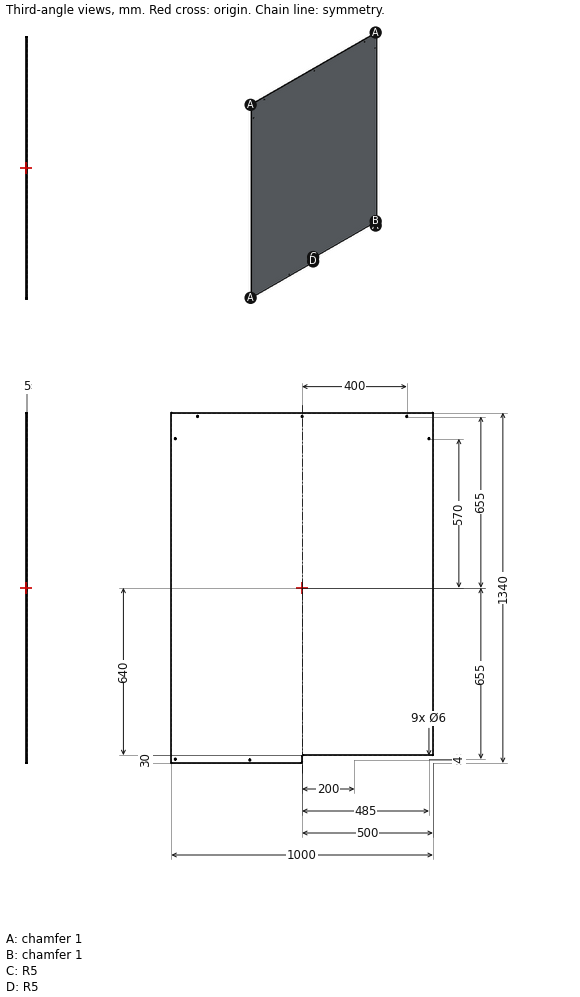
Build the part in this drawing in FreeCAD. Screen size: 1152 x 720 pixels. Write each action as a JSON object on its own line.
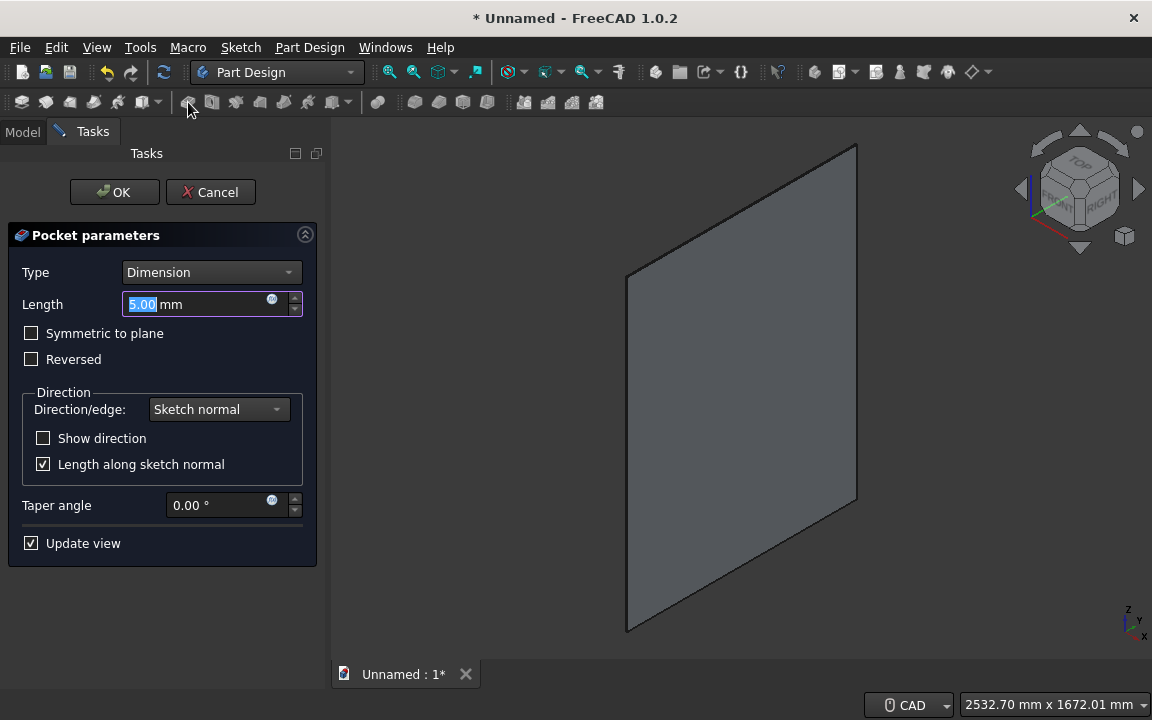
{"action": "left_click", "coordinate": [212, 272]}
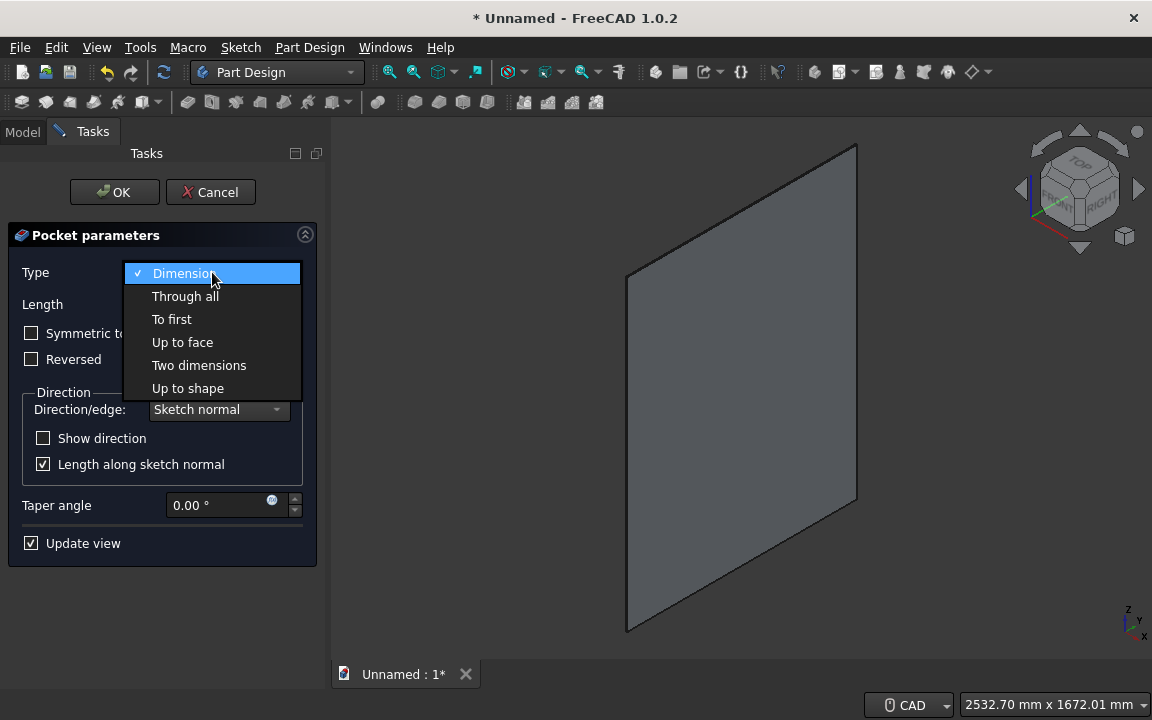
{"action": "left_click", "coordinate": [212, 296]}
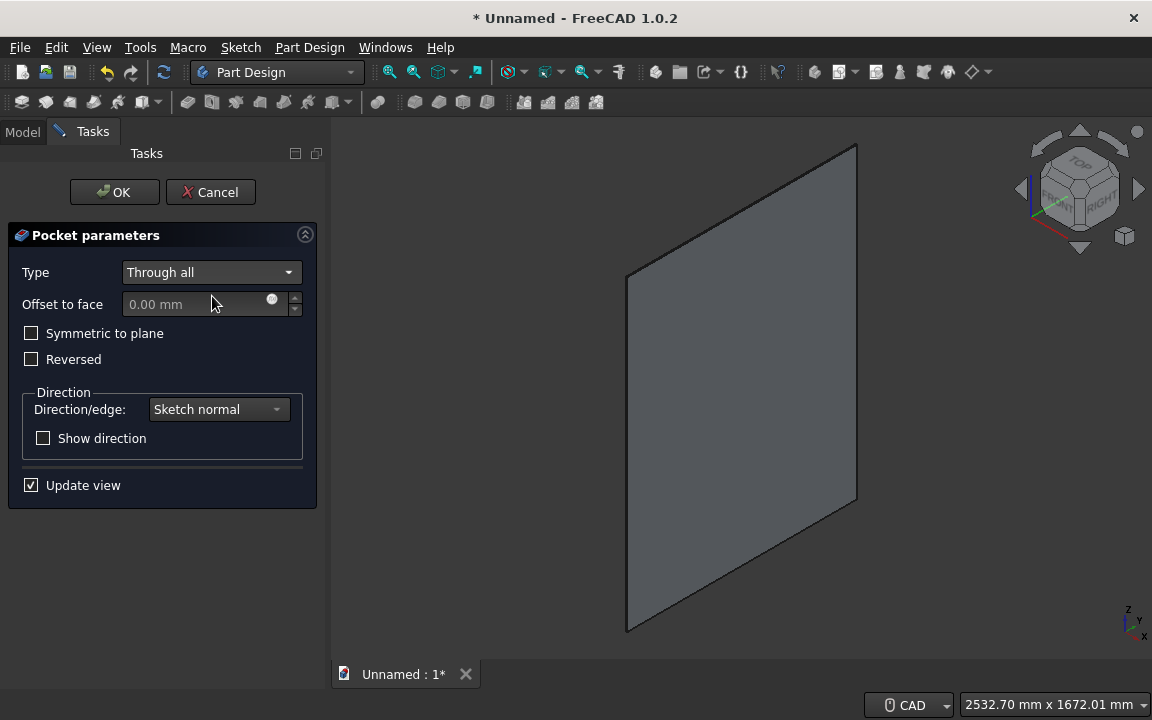
{"action": "left_click", "coordinate": [30, 359]}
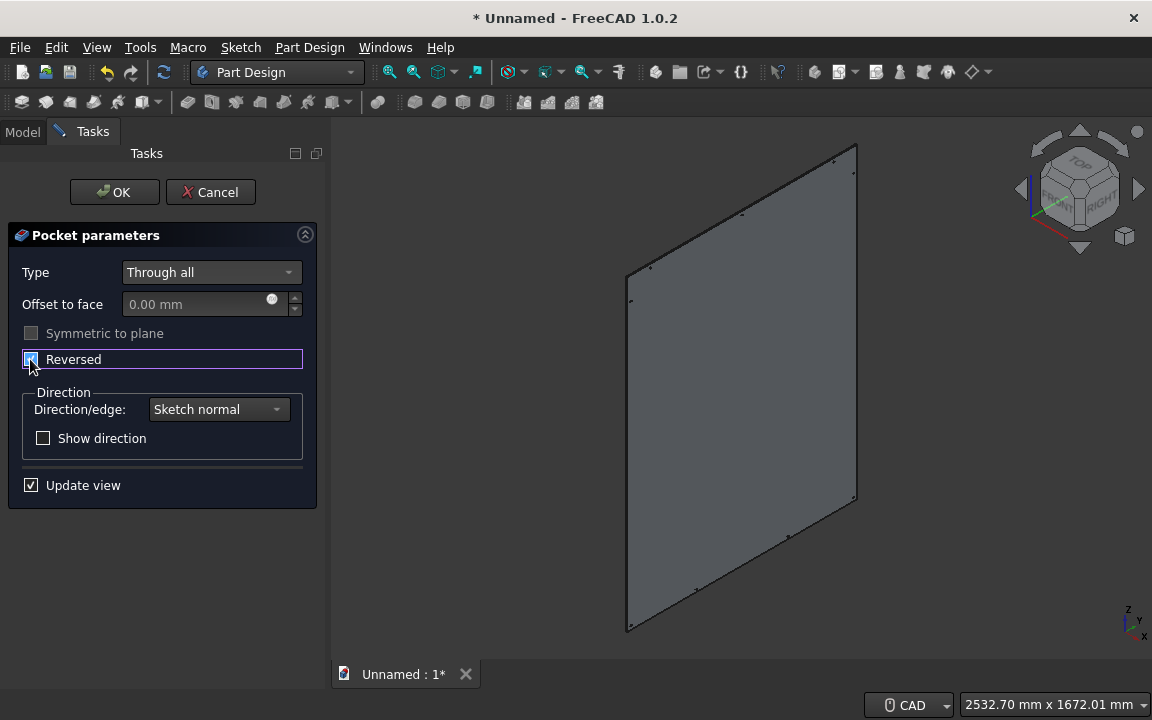
{"action": "left_click", "coordinate": [115, 192]}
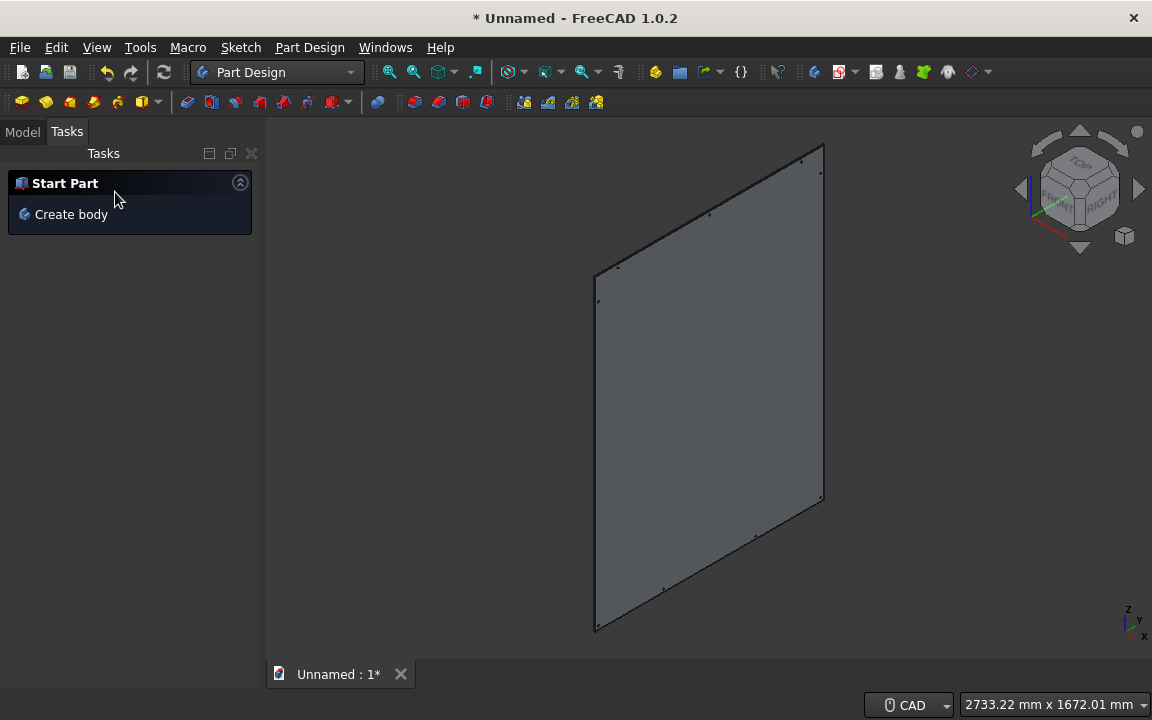
{"action": "left_click", "coordinate": [710, 387]}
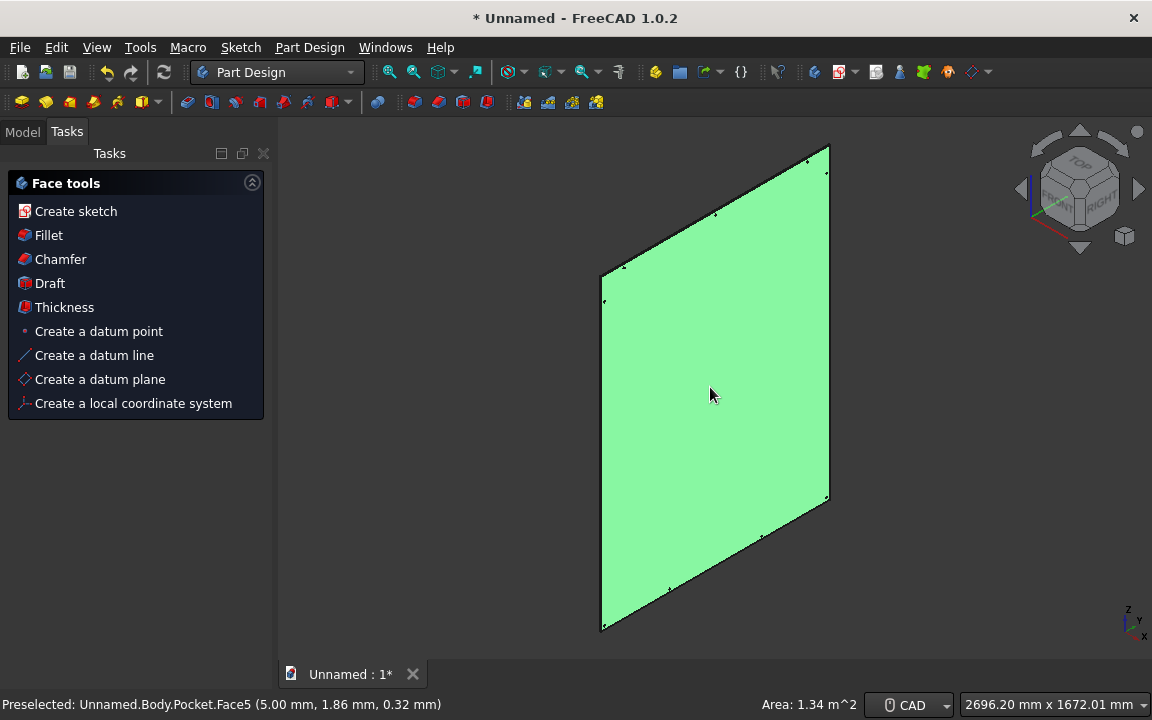
{"action": "left_click", "coordinate": [840, 72]}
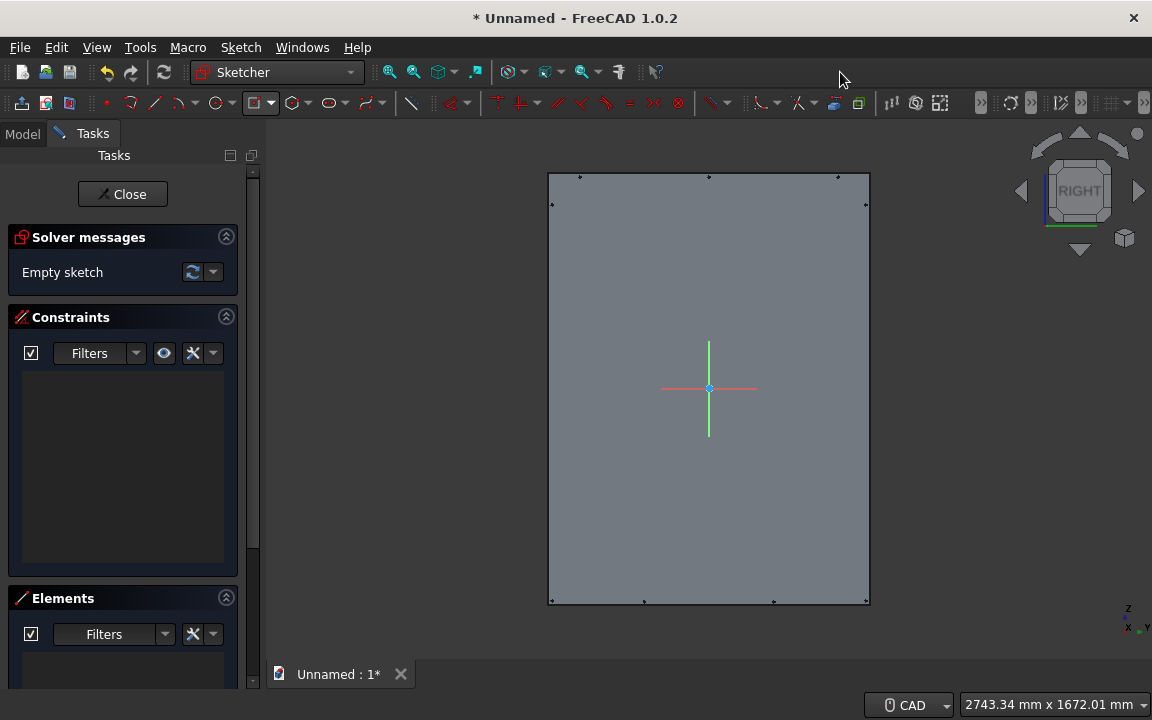
{"action": "scroll", "coordinate": [987, 631], "scroll_direction": "up", "scroll_amount": 2}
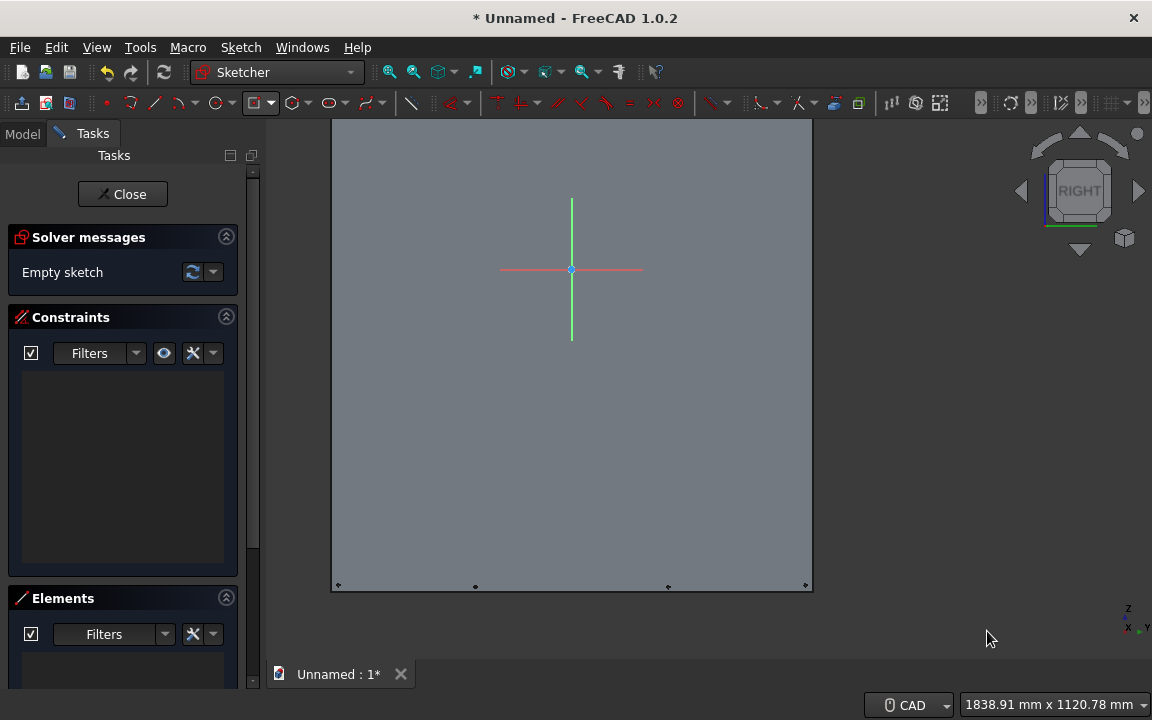
{"action": "key", "text": "g r"}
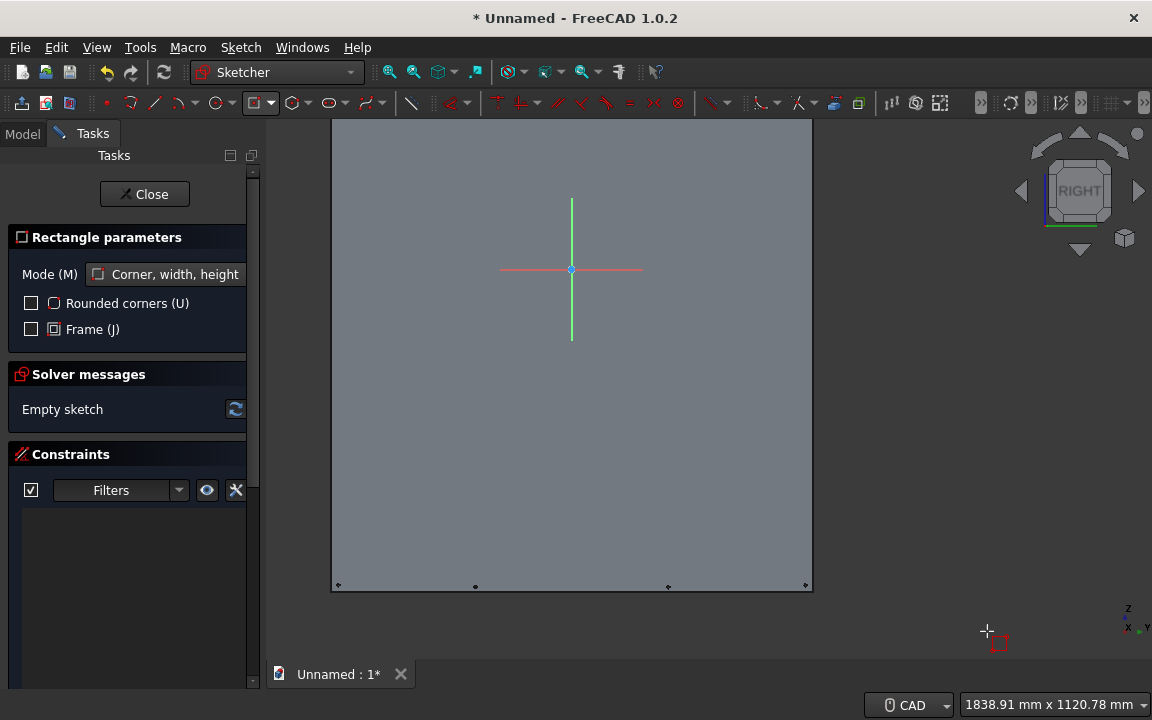
{"action": "left_click", "coordinate": [572, 578]}
{"action": "left_click", "coordinate": [813, 592]}
{"action": "key", "text": "Escape"}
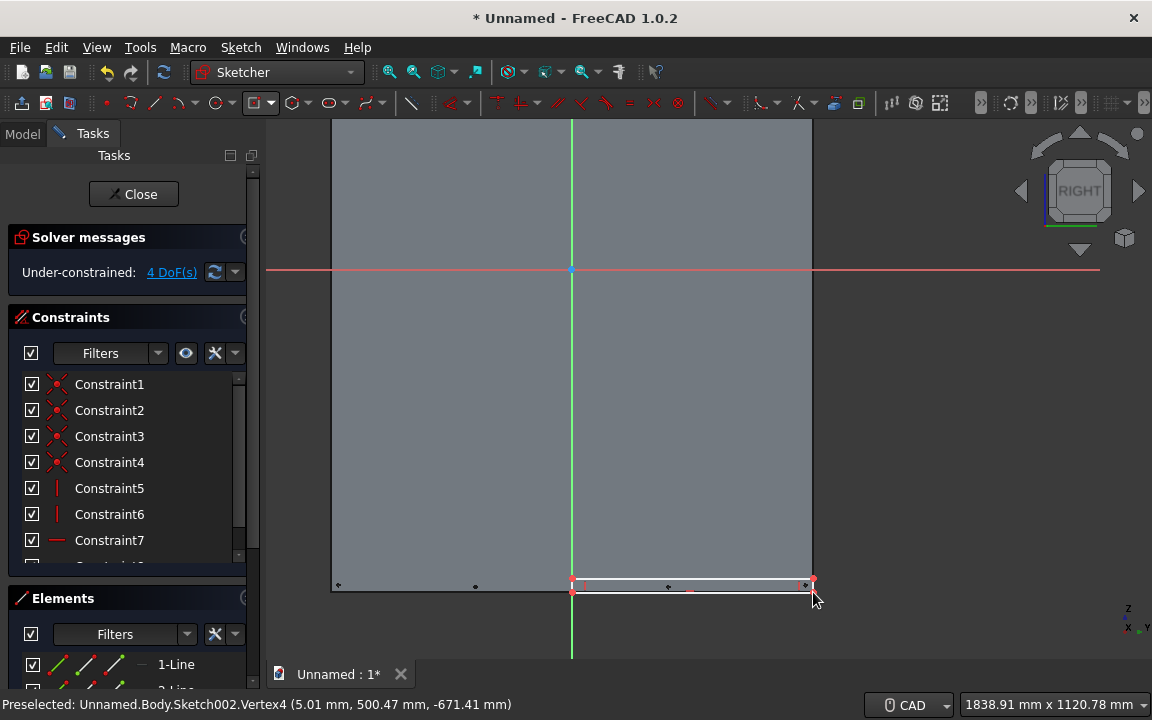
{"action": "left_click", "coordinate": [572, 579]}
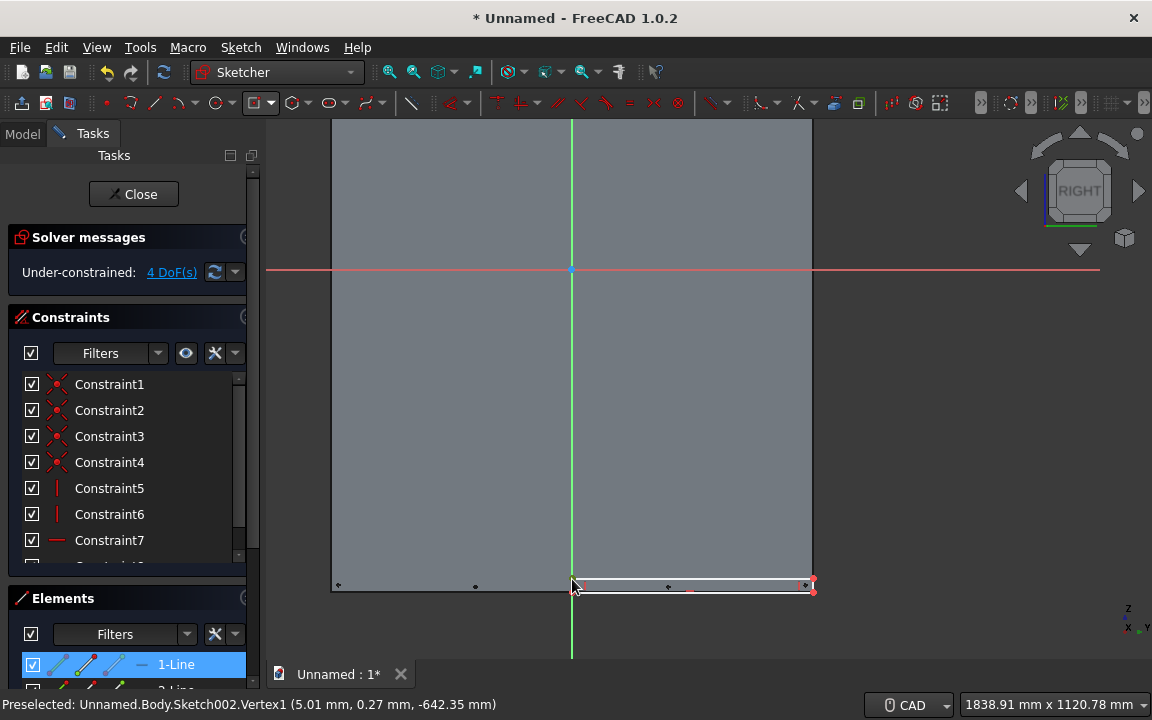
{"action": "left_click", "coordinate": [572, 527]}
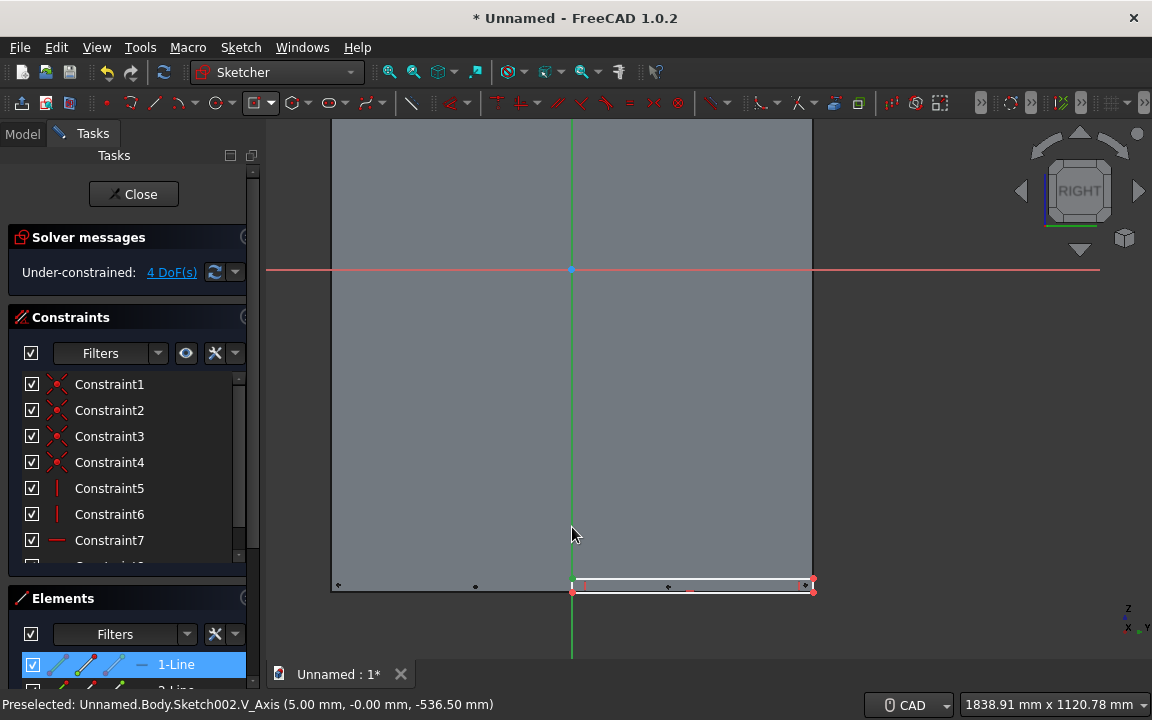
{"action": "left_click", "coordinate": [498, 104]}